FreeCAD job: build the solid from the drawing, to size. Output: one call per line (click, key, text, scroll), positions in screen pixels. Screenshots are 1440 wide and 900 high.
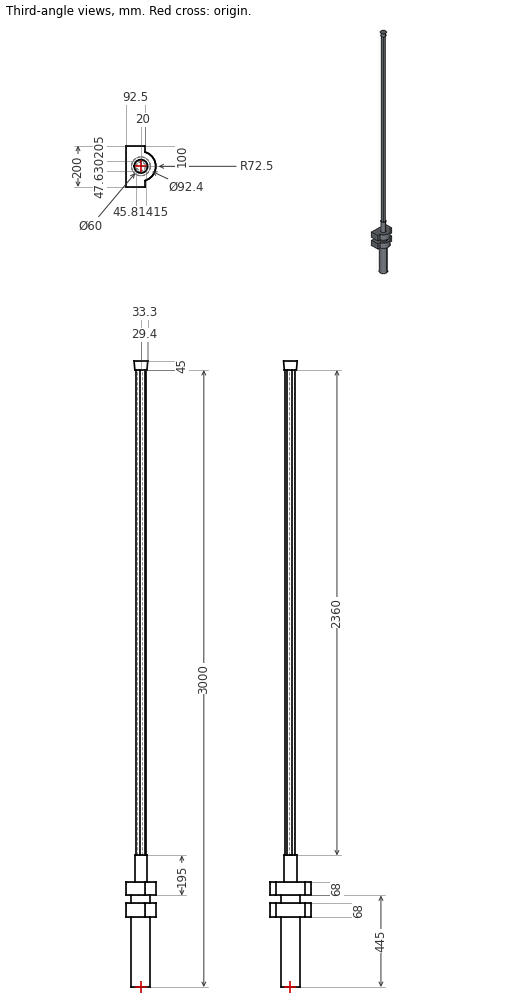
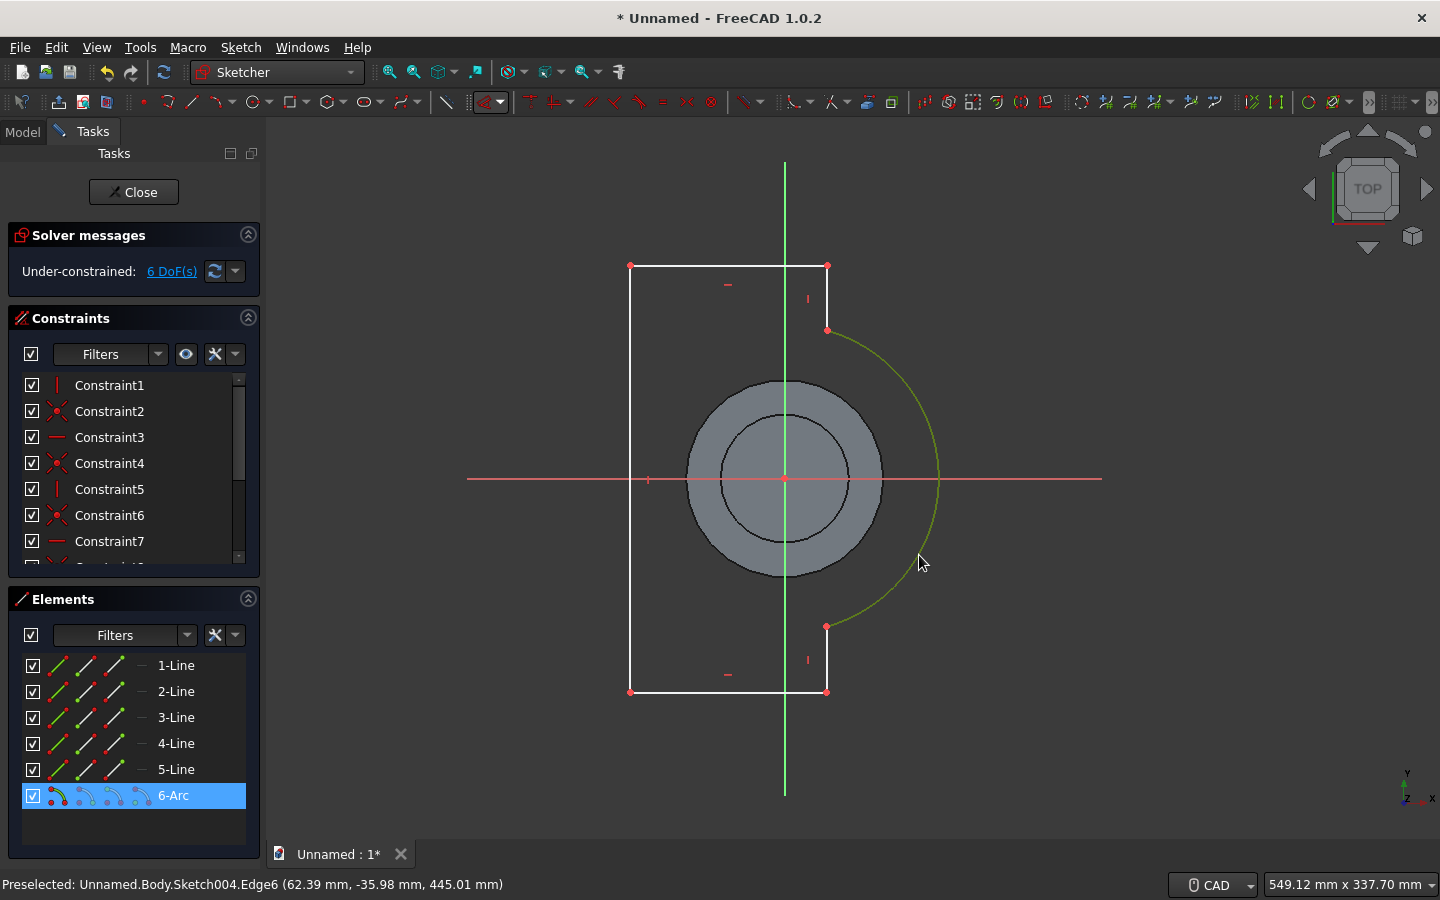
key(k)
key(r)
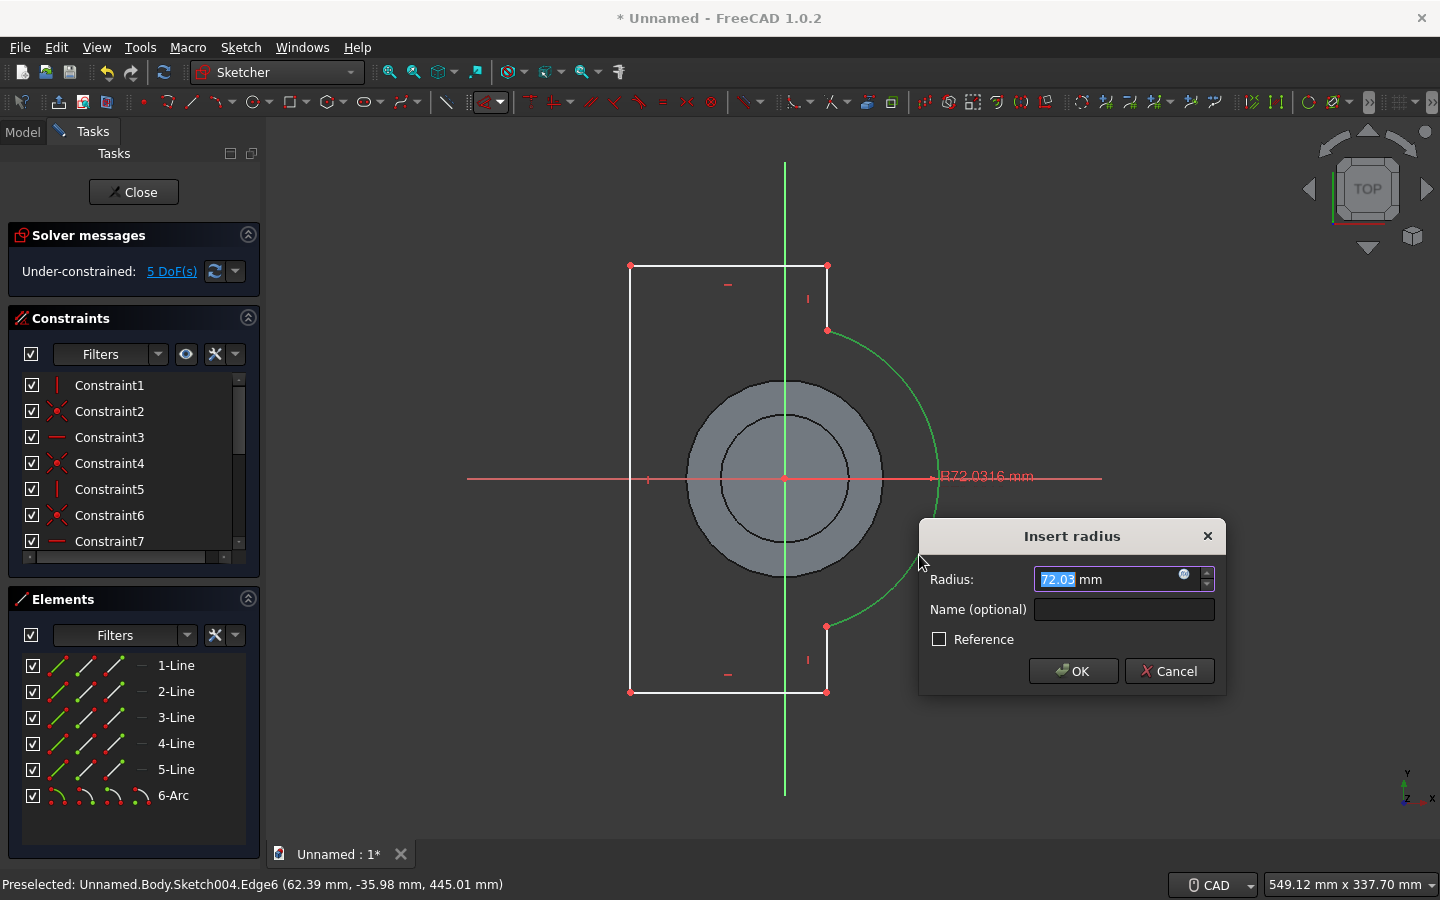
text(72.5)
key(Return)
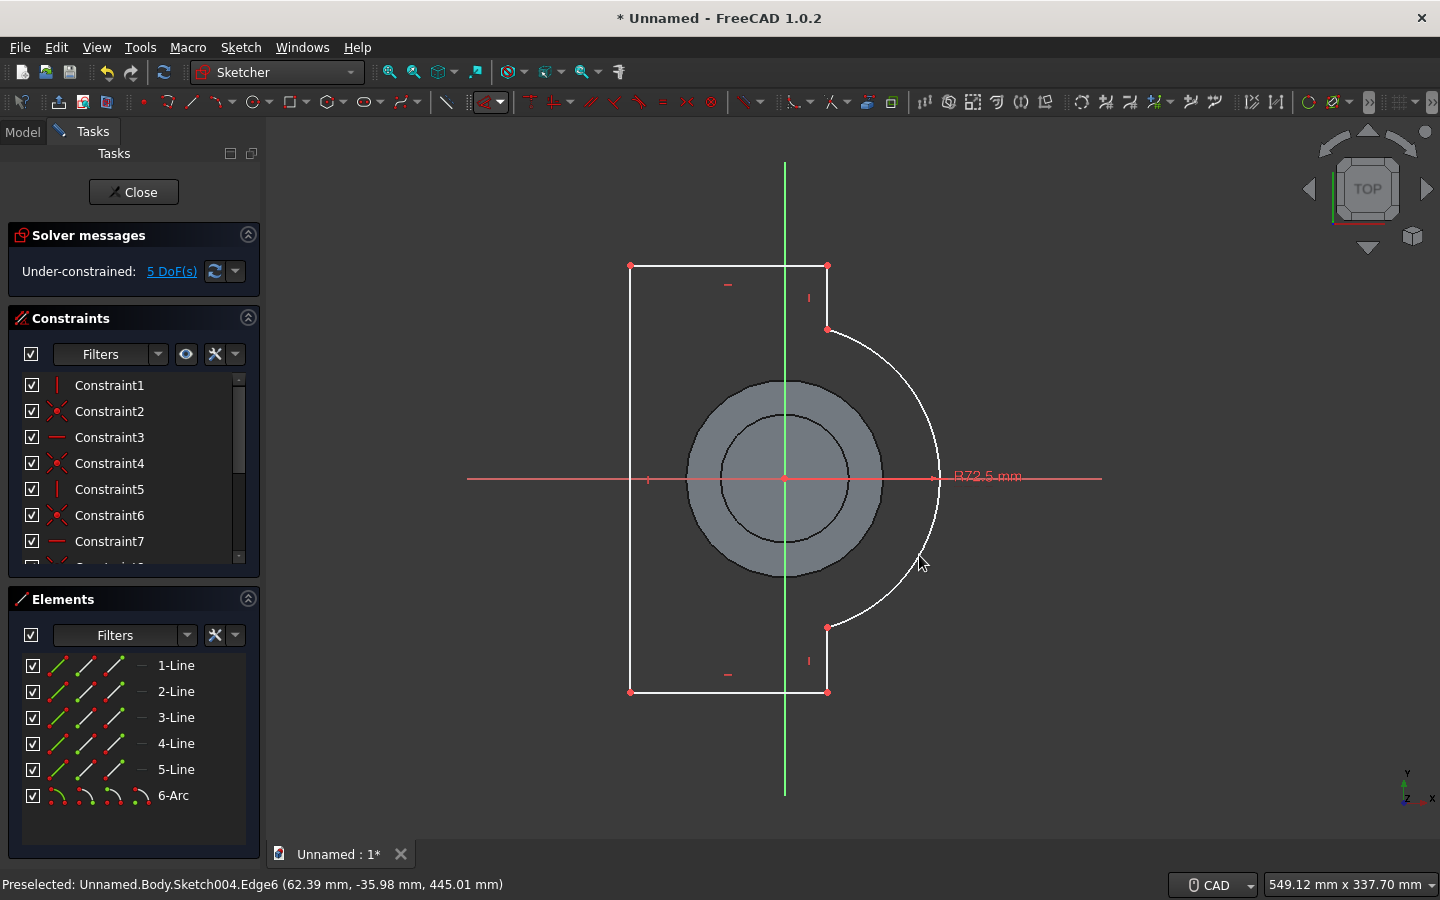
click(630, 394)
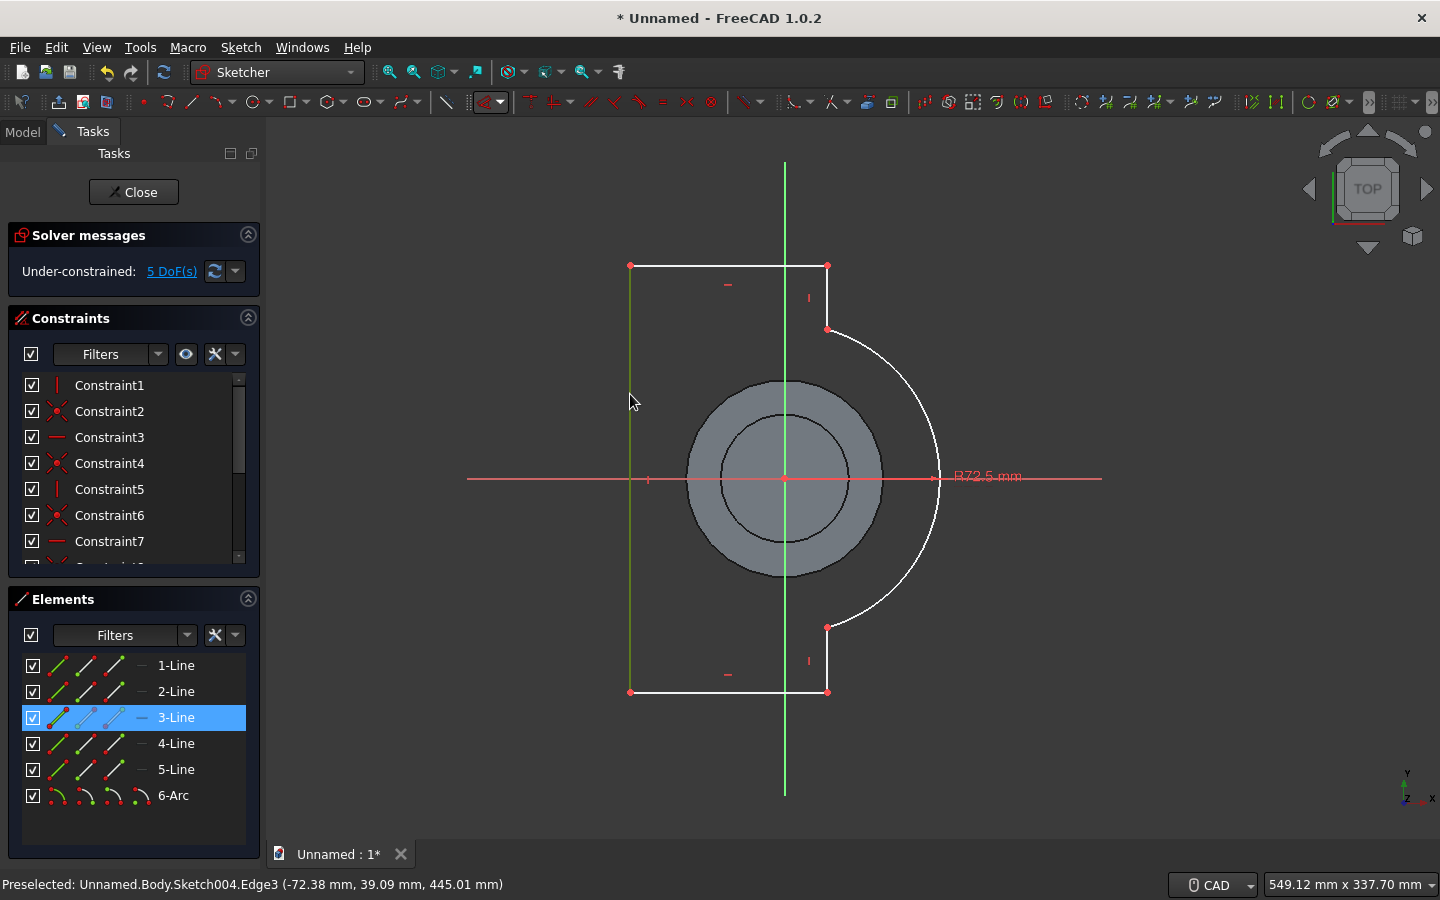
key(i)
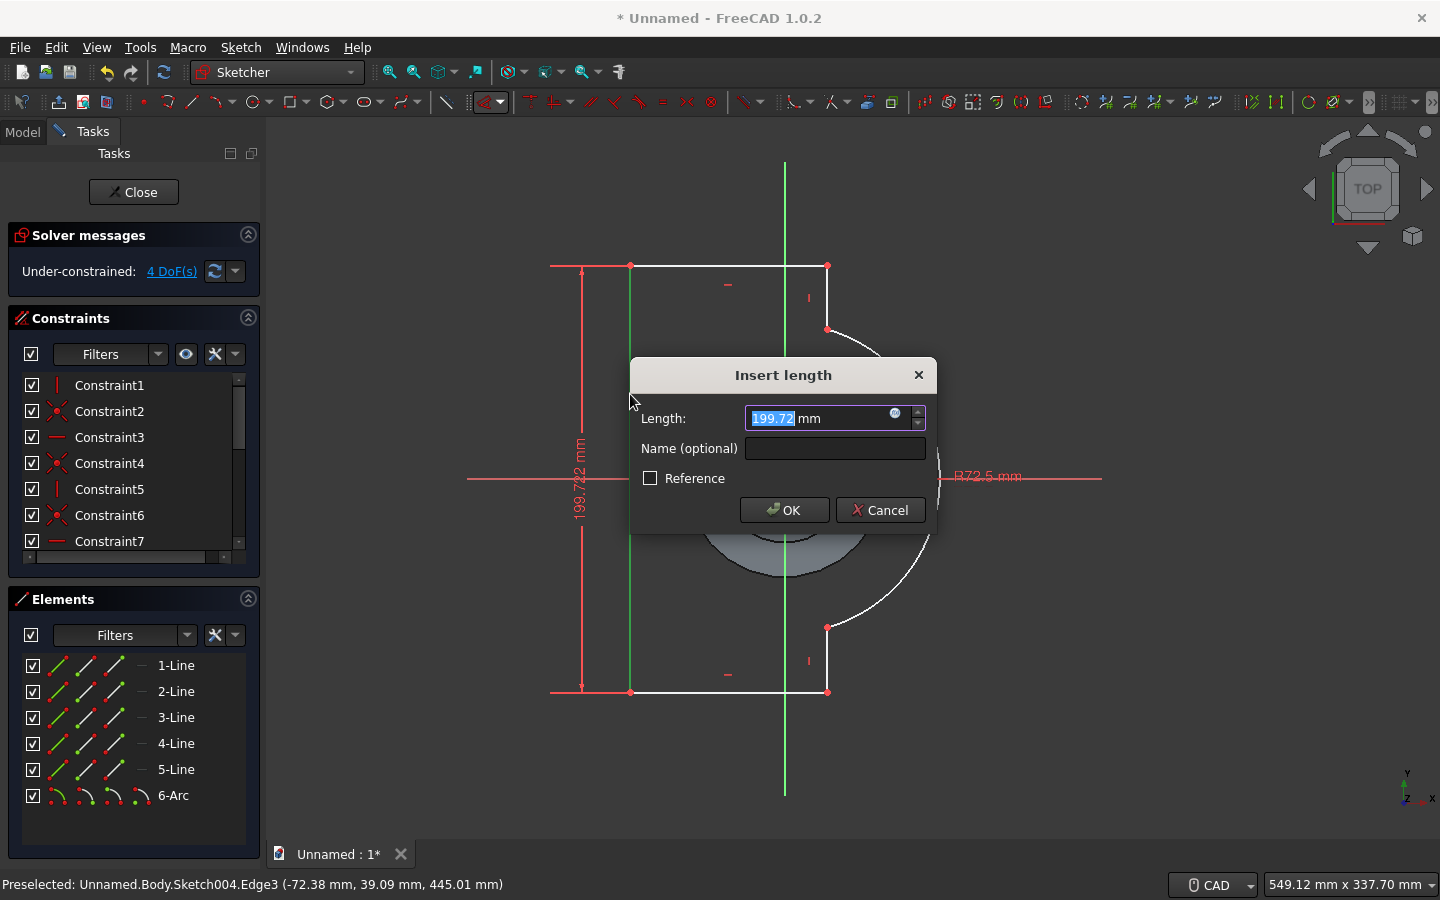
text(200)
key(Return)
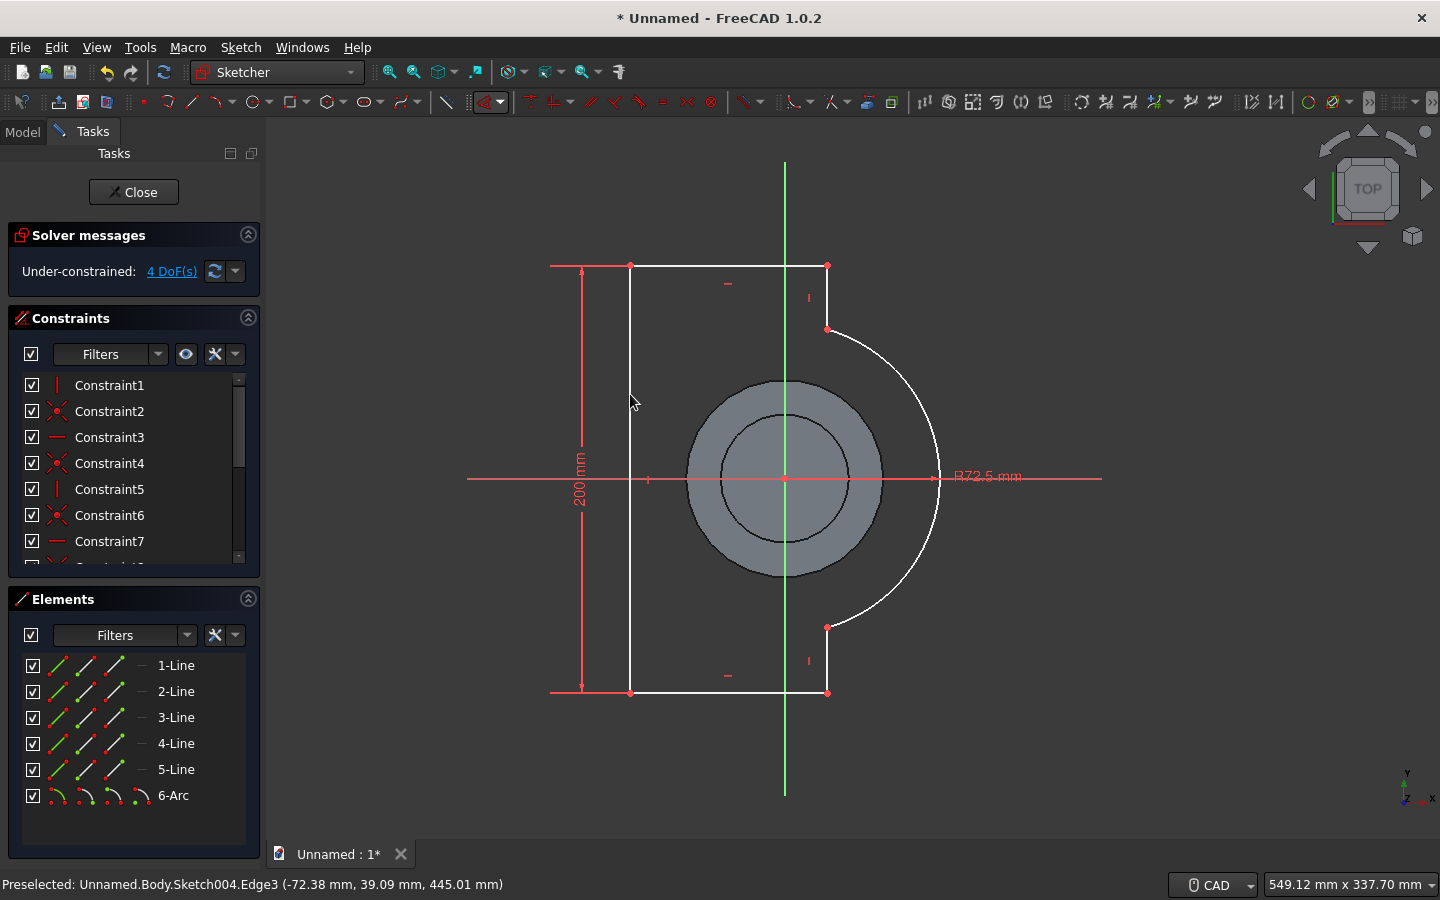
click(827, 329)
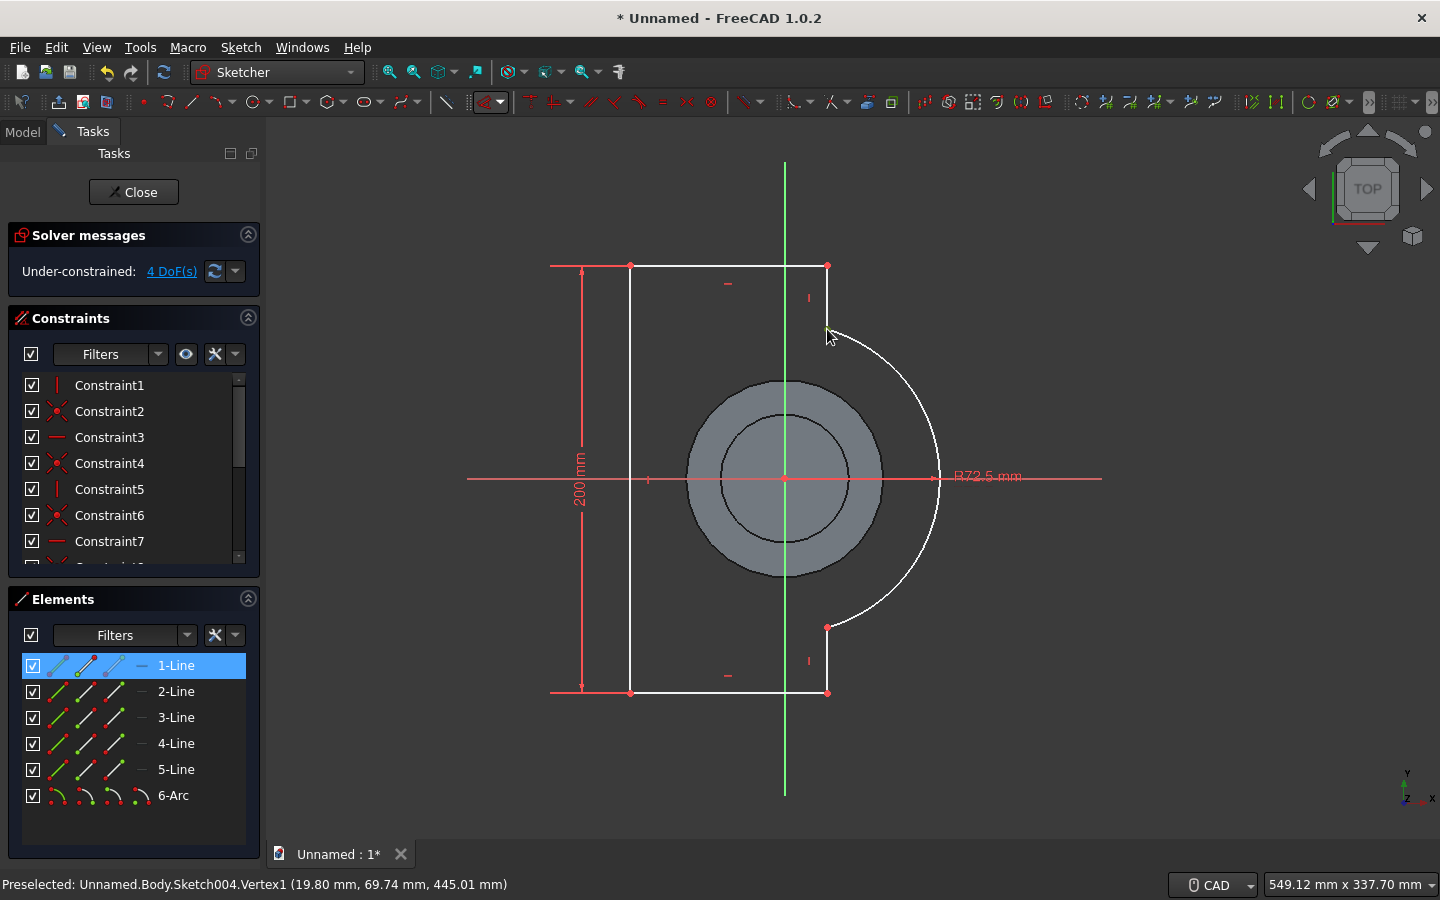
click(502, 102)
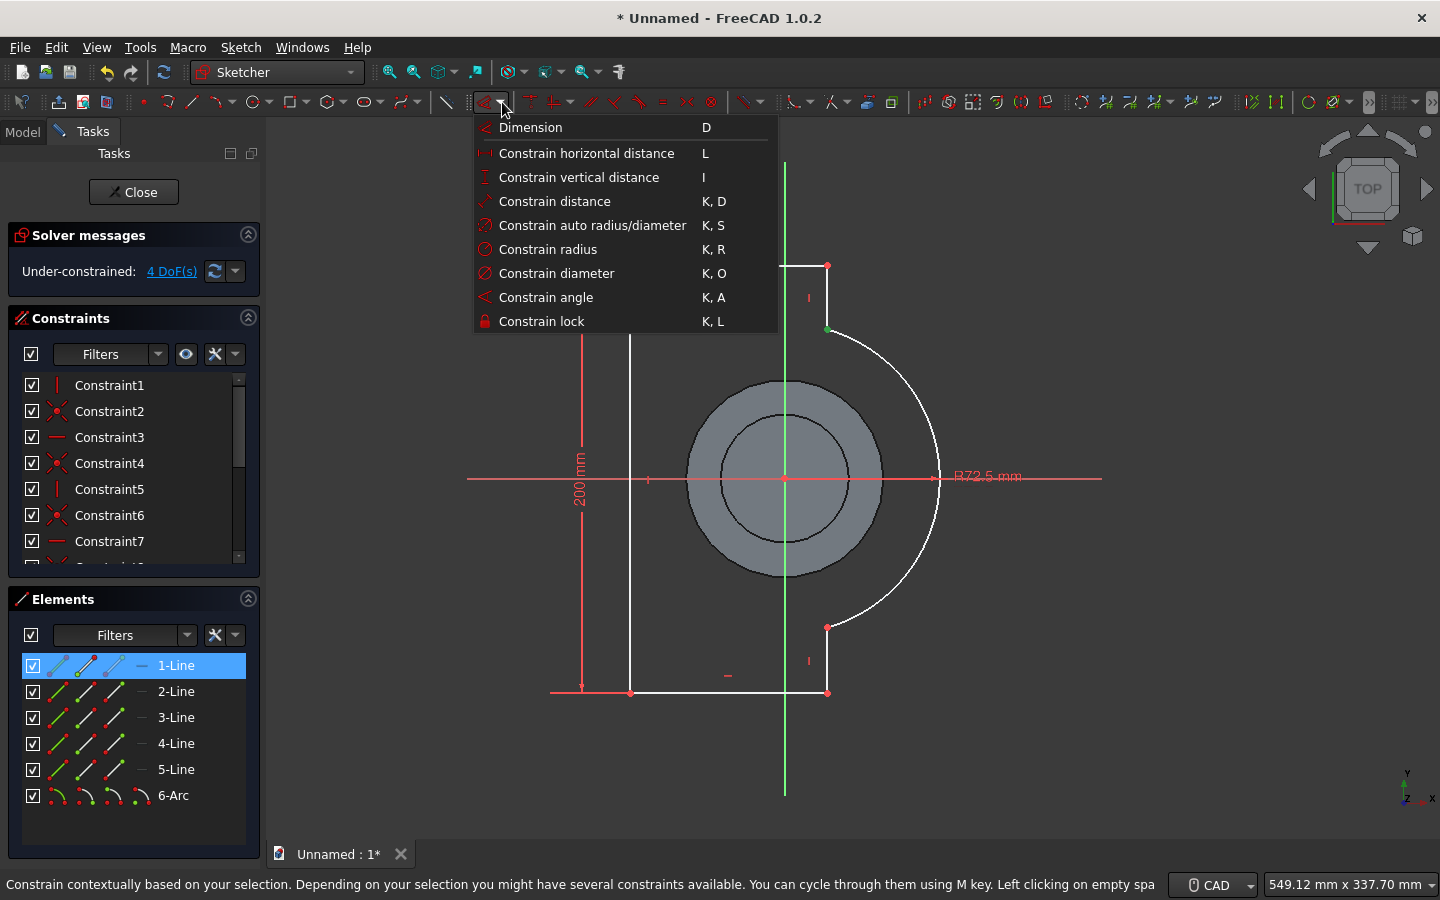
click(626, 153)